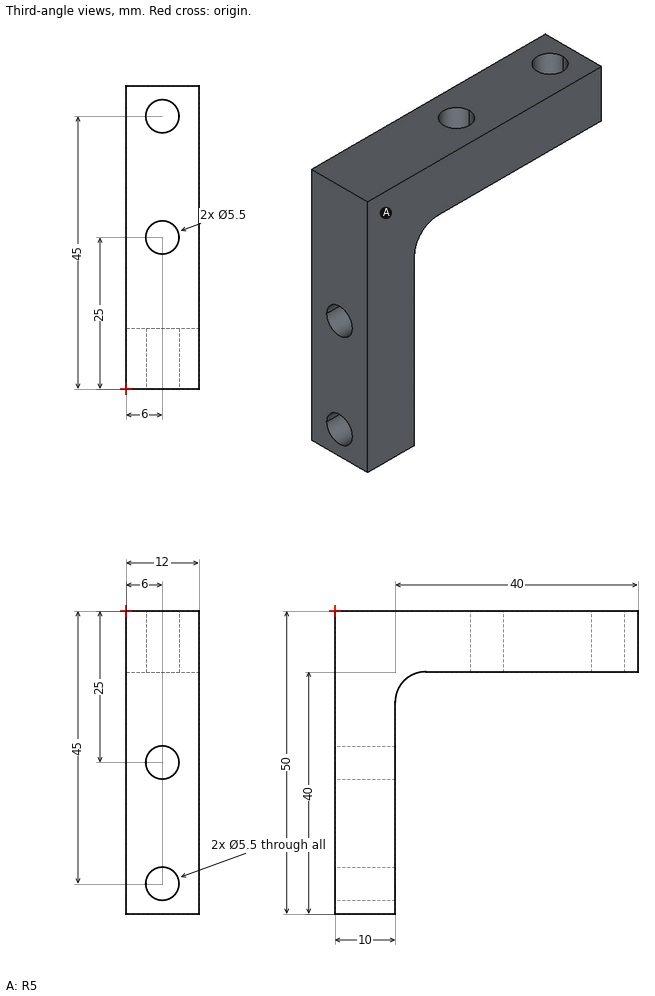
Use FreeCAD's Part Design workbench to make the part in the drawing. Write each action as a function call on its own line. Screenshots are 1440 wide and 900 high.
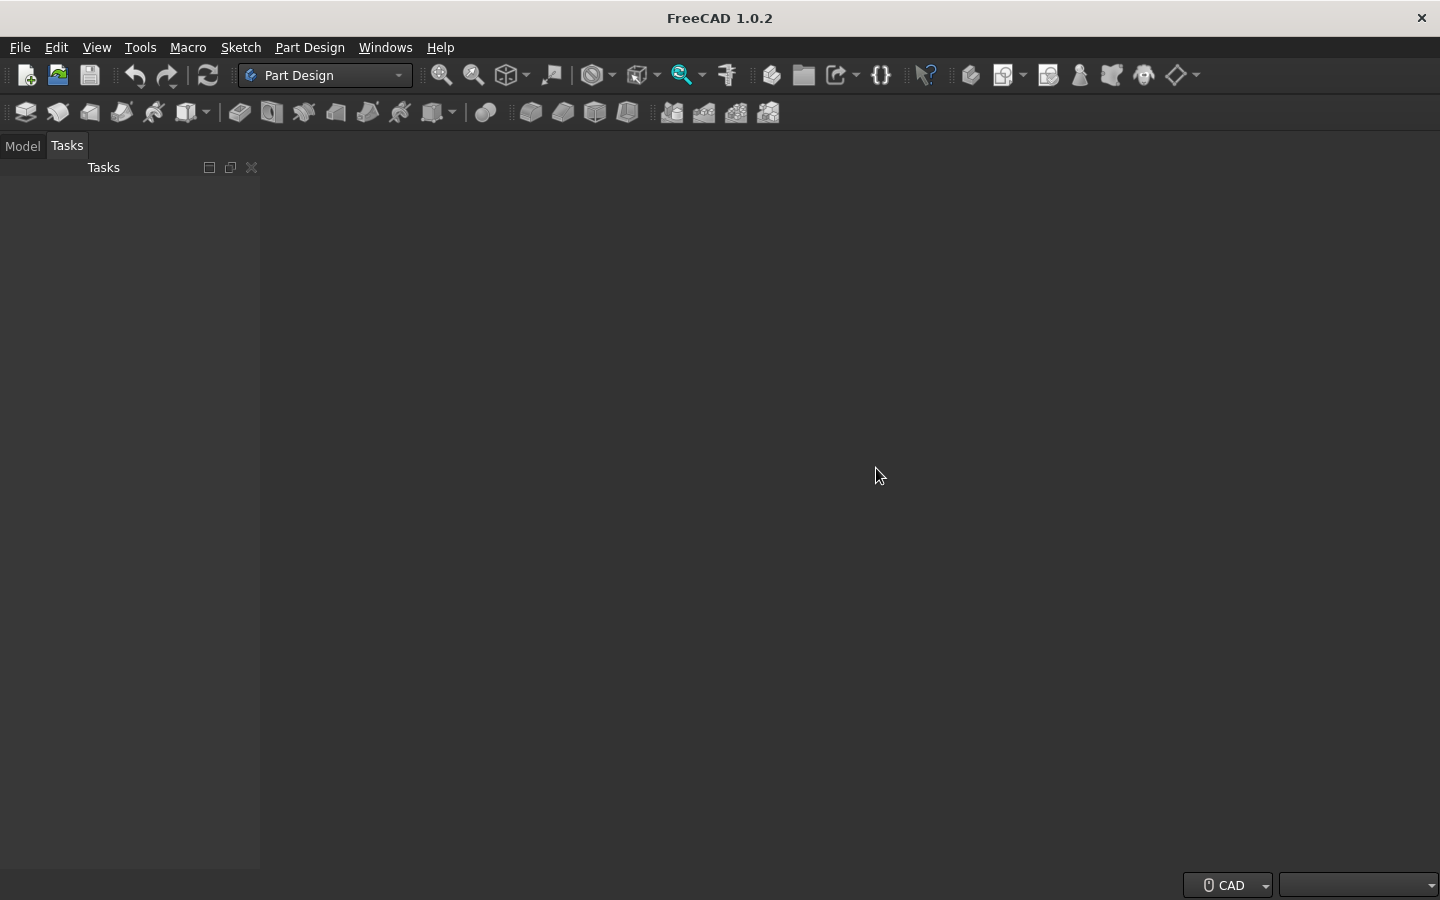
click(26, 76)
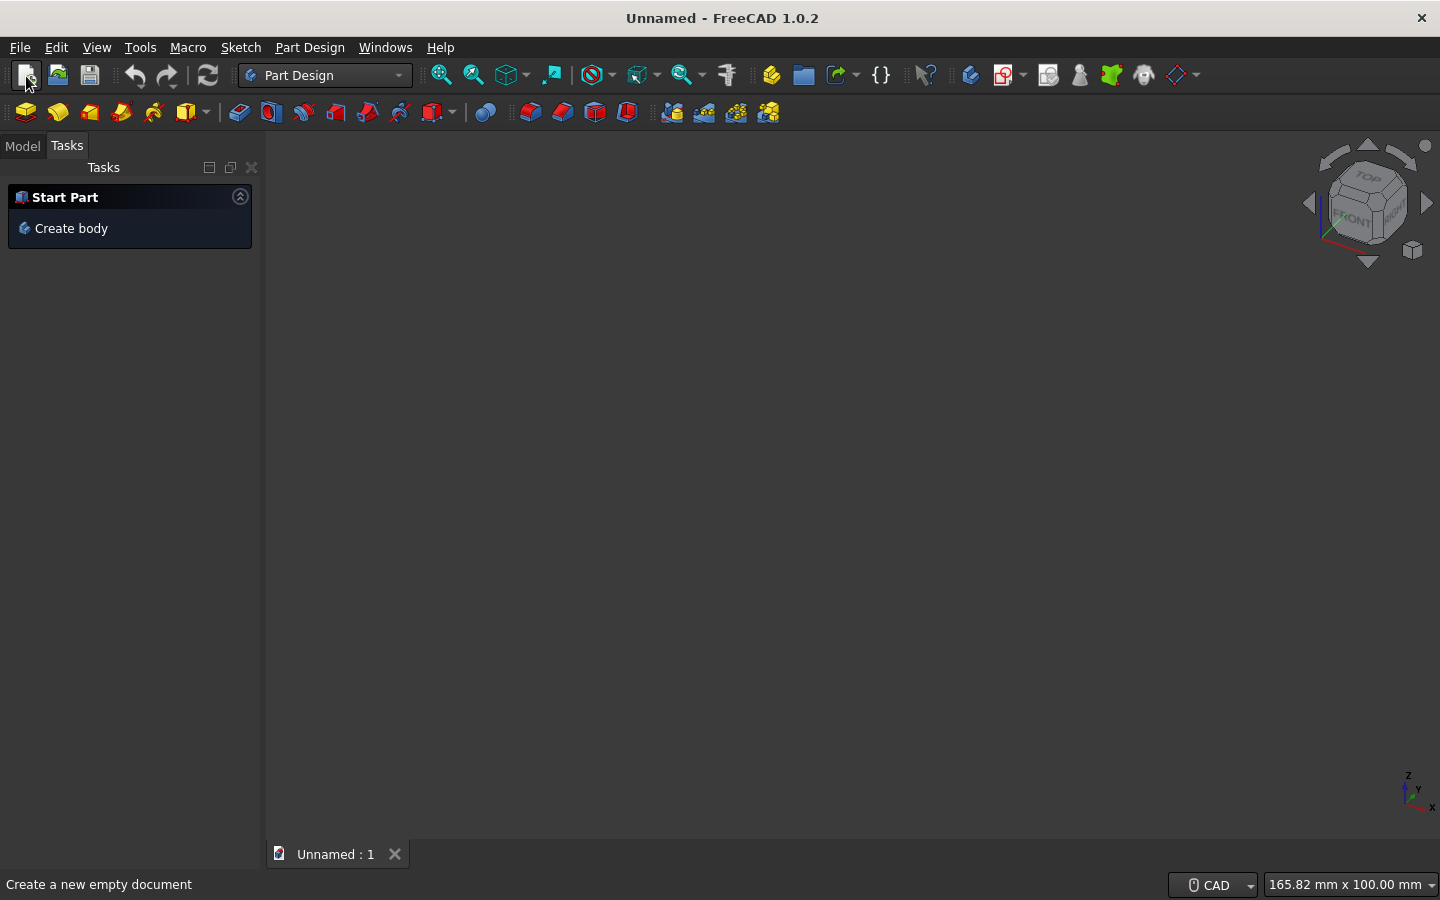
click(1004, 76)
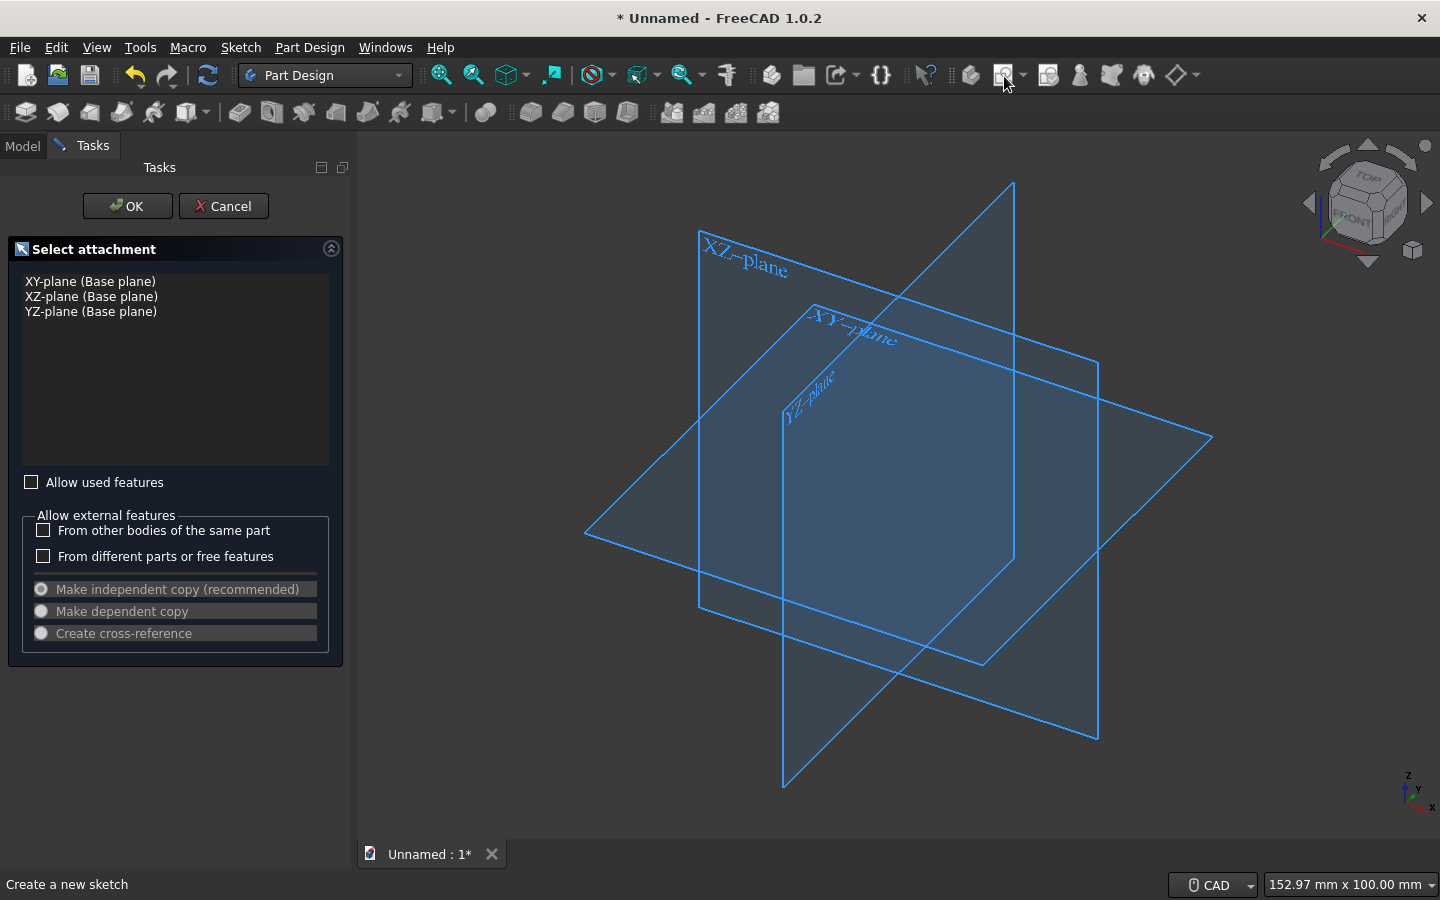
click(82, 312)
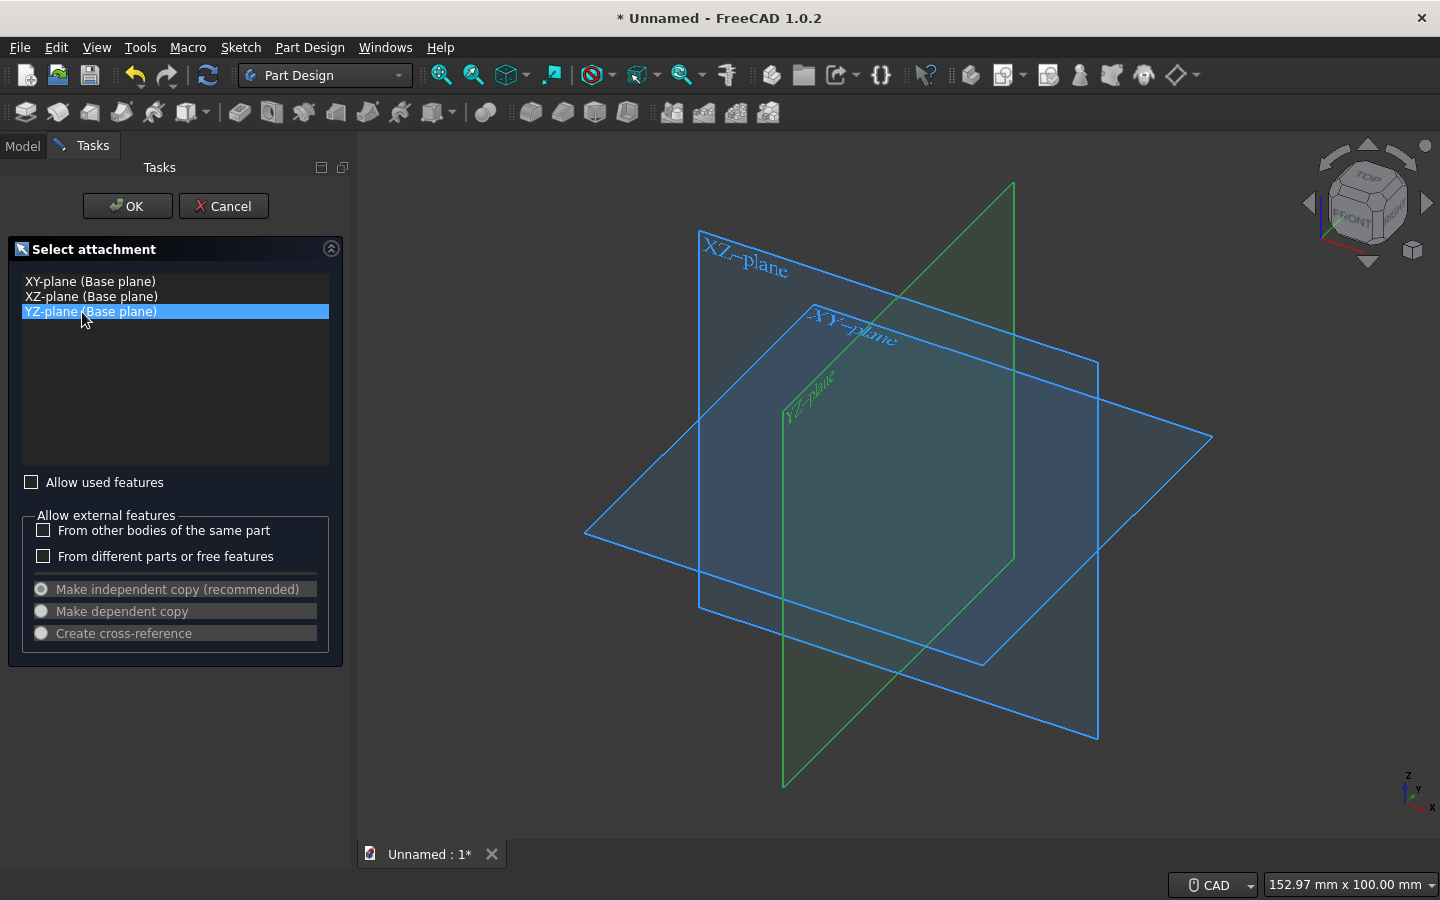
click(128, 206)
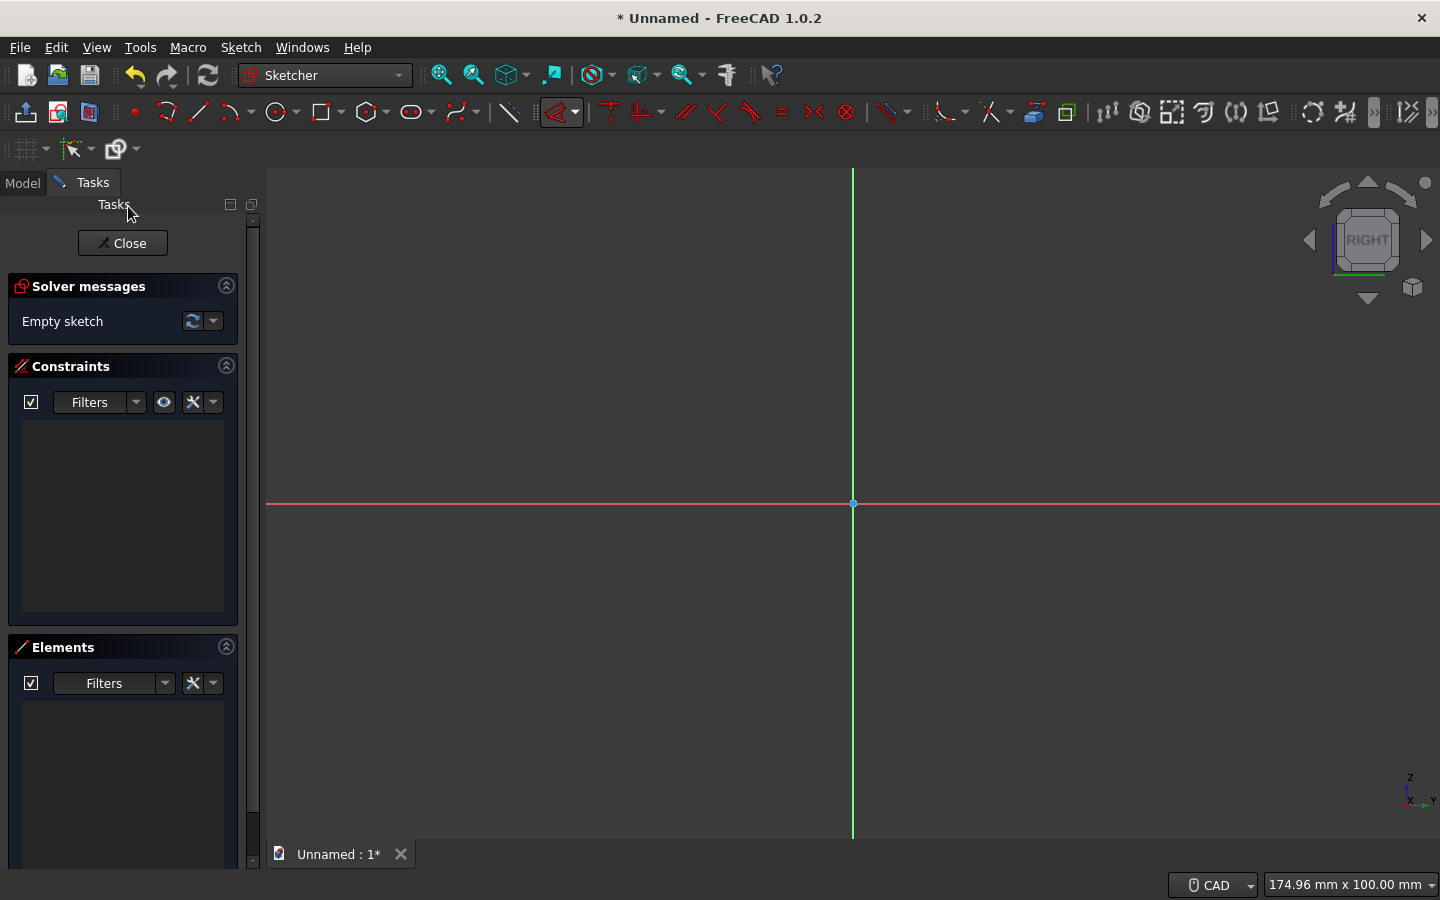
scroll(294, 196, down, 1)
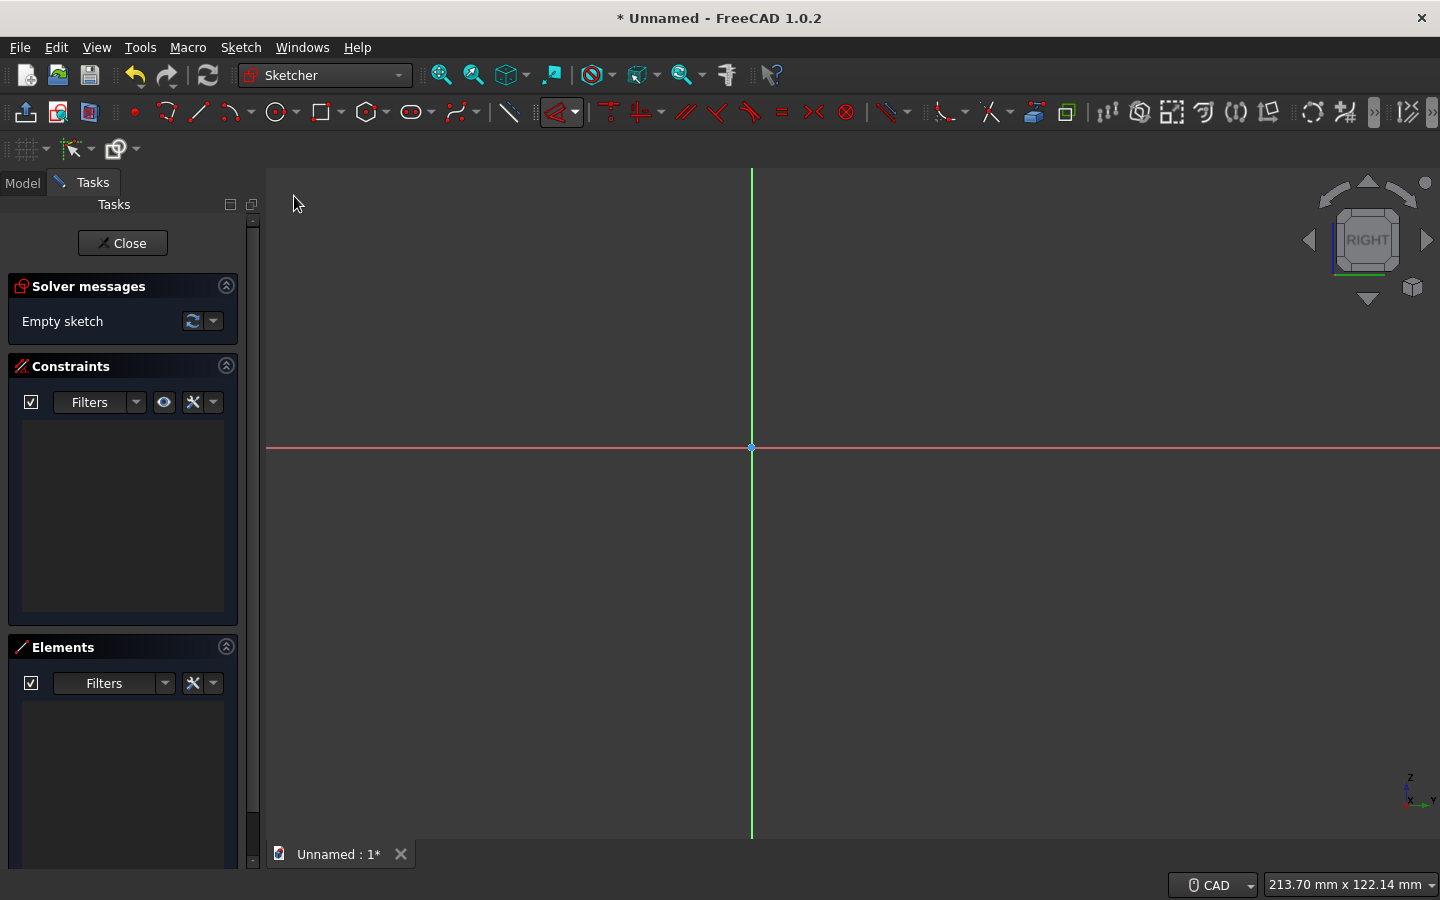
scroll(1102, 751, up, 2)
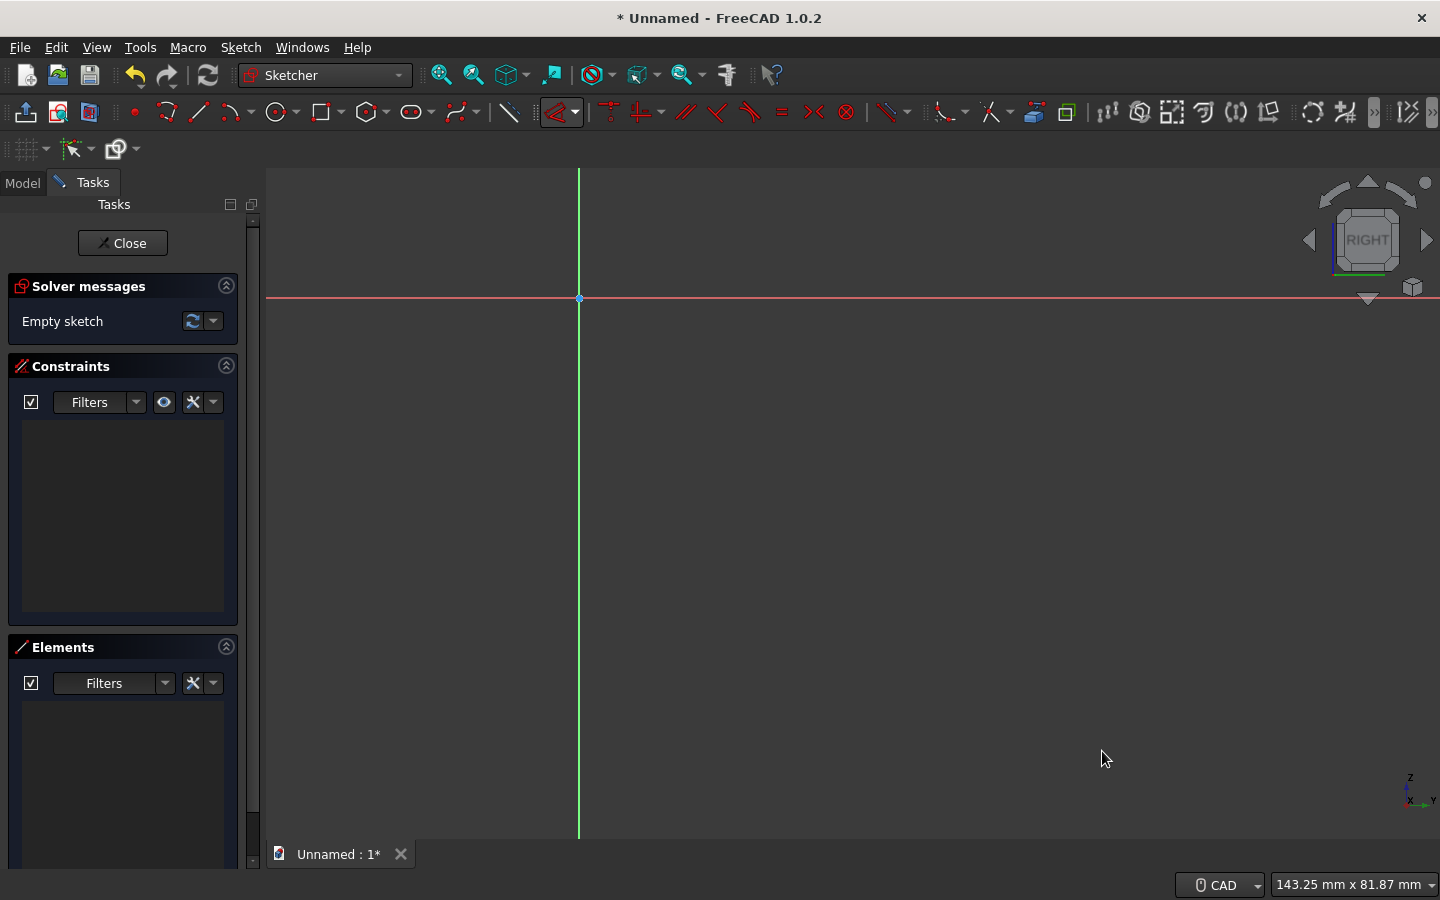
click(168, 112)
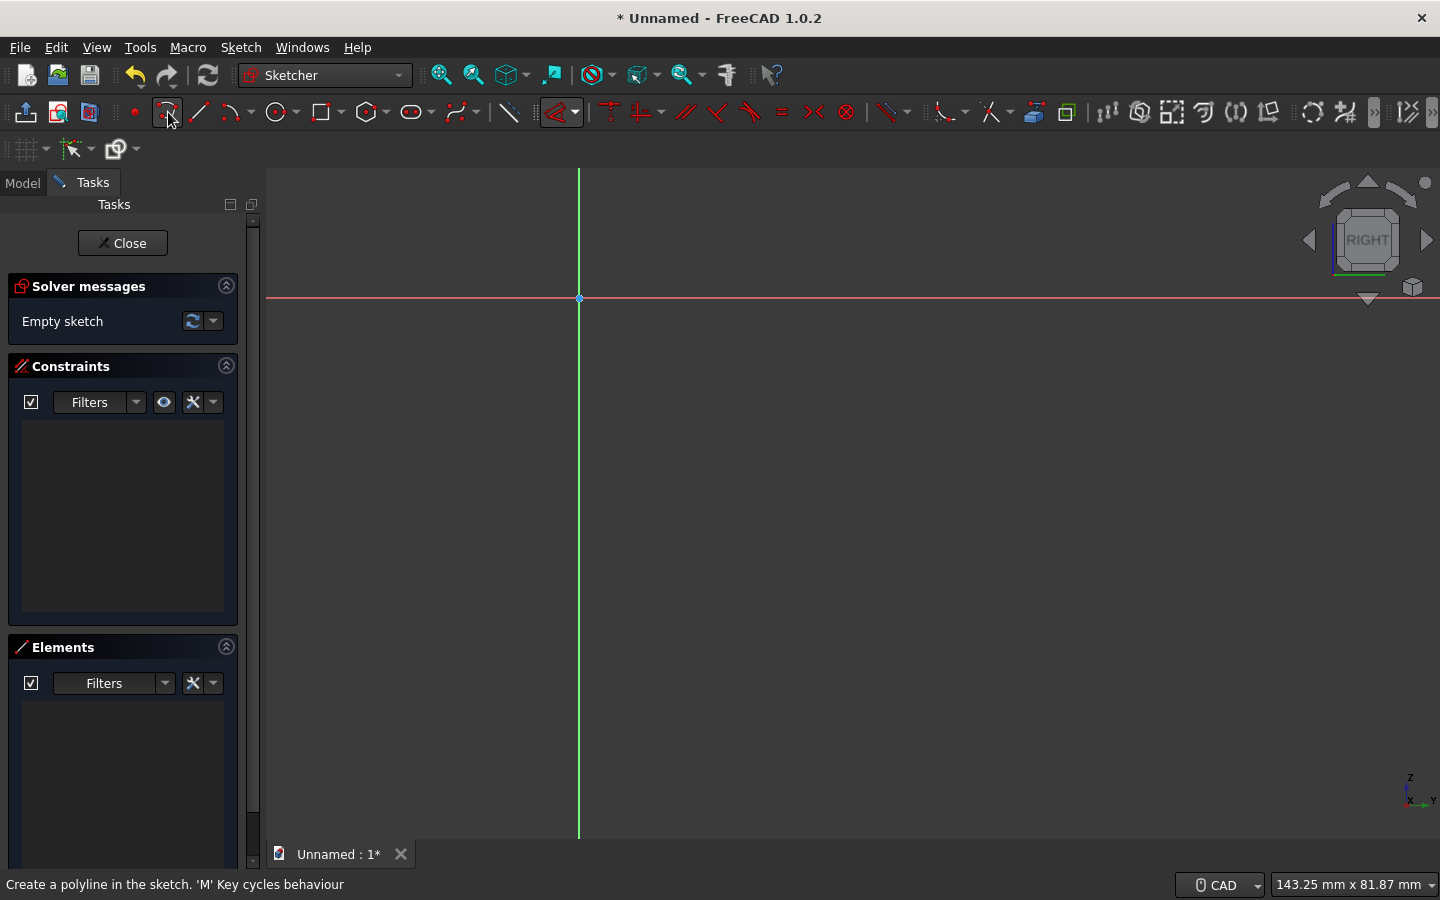
click(579, 298)
click(588, 708)
click(661, 708)
click(661, 380)
click(989, 380)
click(989, 307)
click(579, 298)
key(Escape)
key(Escape)